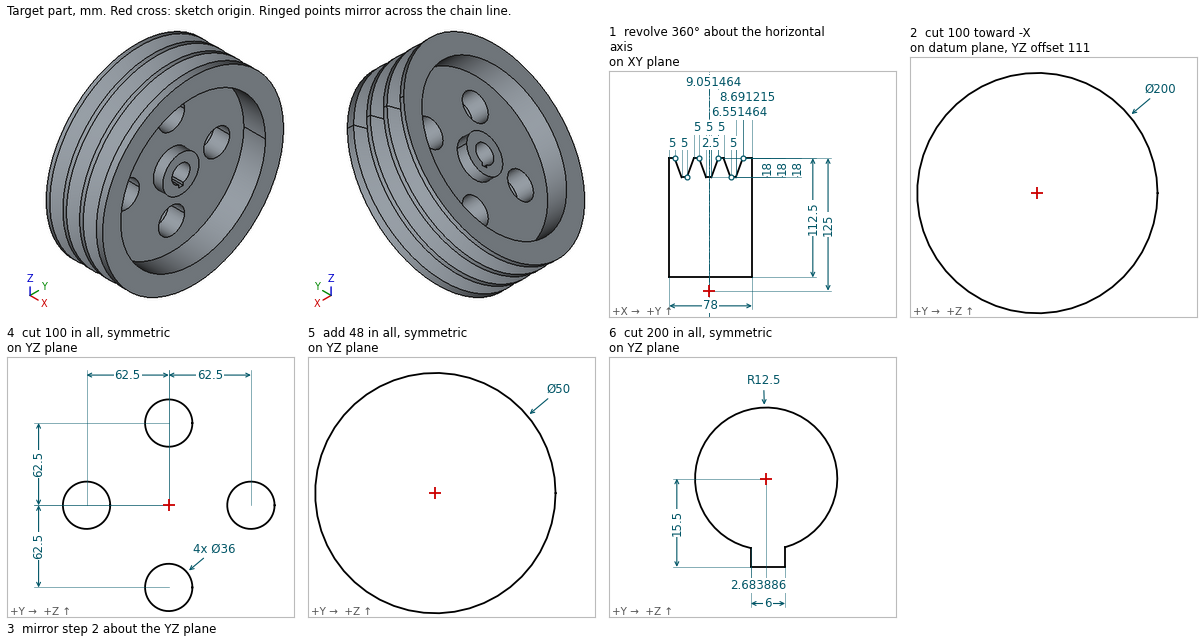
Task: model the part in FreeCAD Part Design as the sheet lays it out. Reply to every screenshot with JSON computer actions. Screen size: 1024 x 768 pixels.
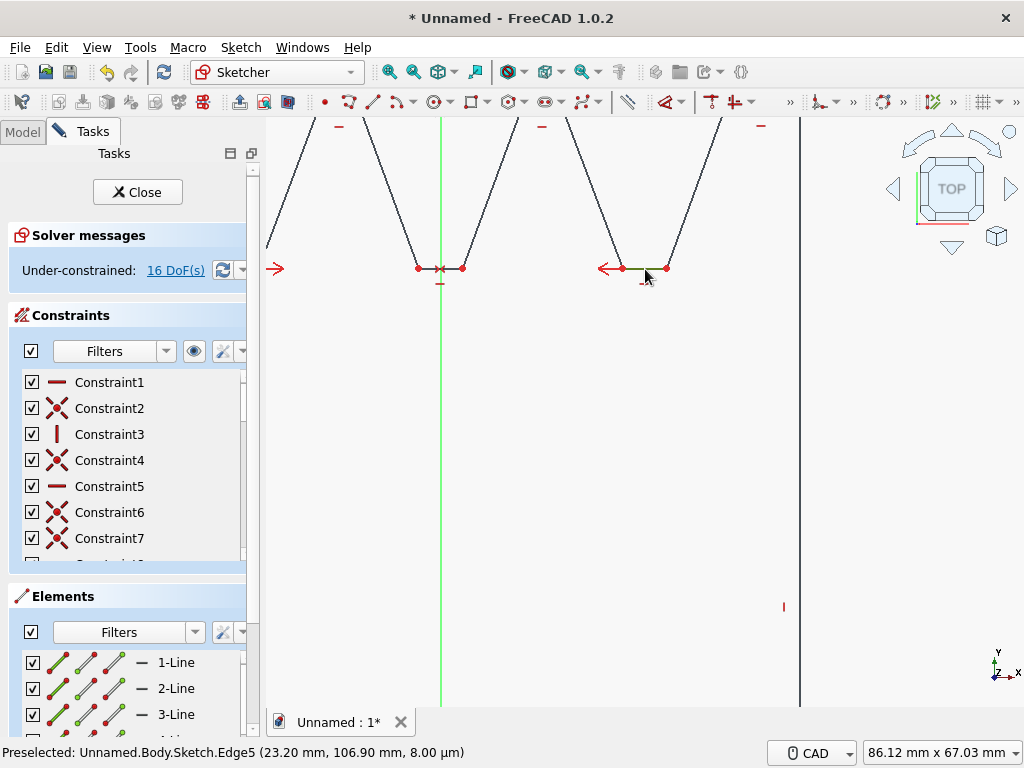
{"action": "left_click", "coordinate": [684, 102]}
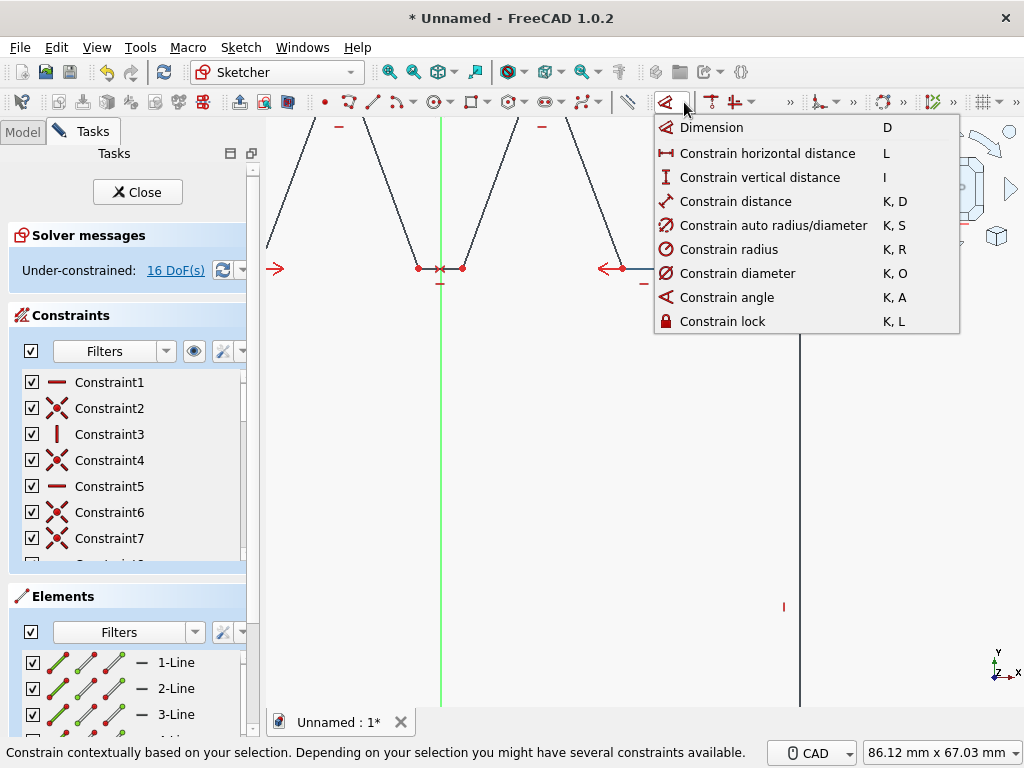
{"action": "left_click", "coordinate": [807, 153]}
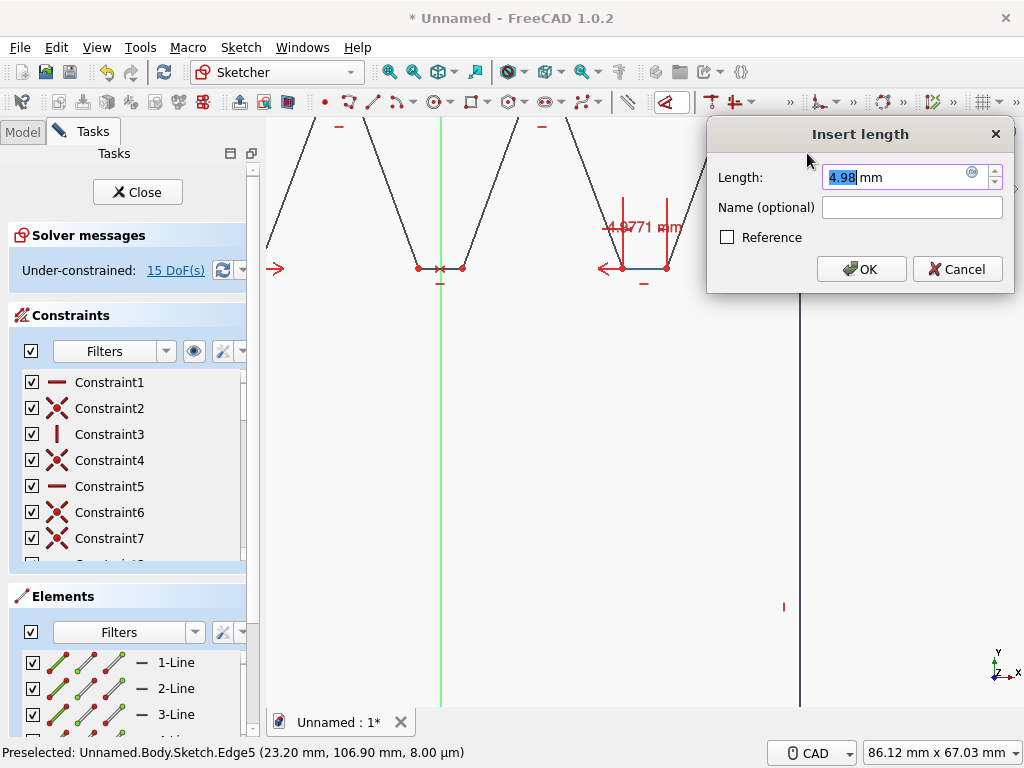
{"action": "type", "text": "5"}
{"action": "key", "text": "Return"}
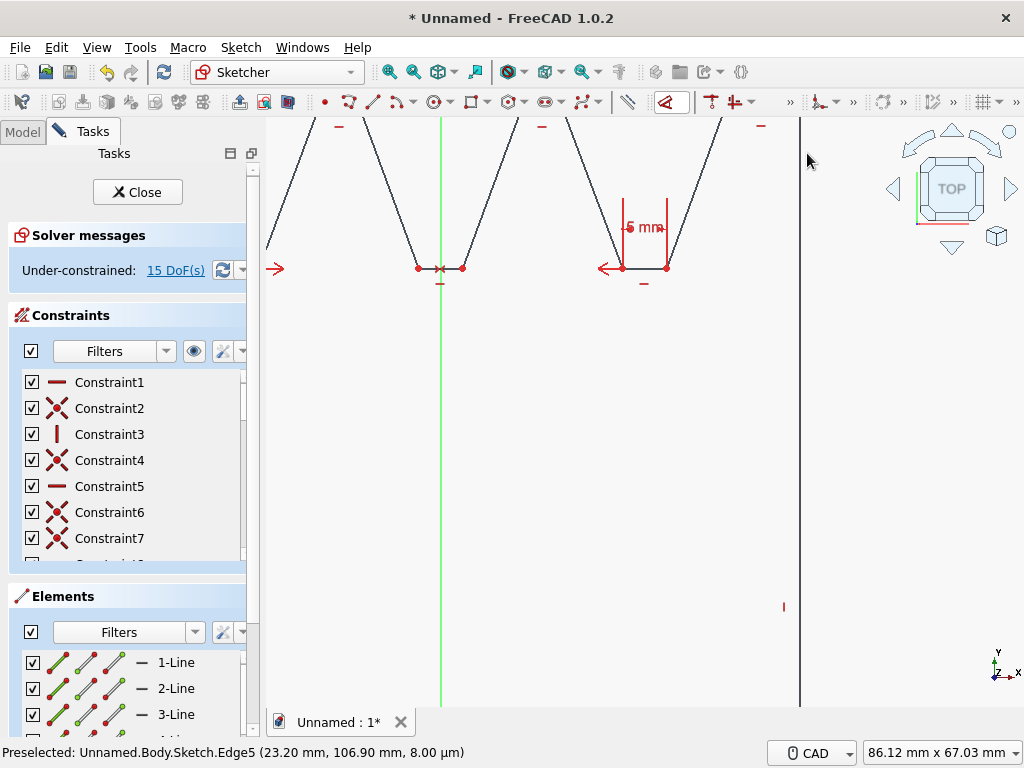
{"action": "scroll", "coordinate": [646, 268], "scroll_direction": "down", "scroll_amount": 5}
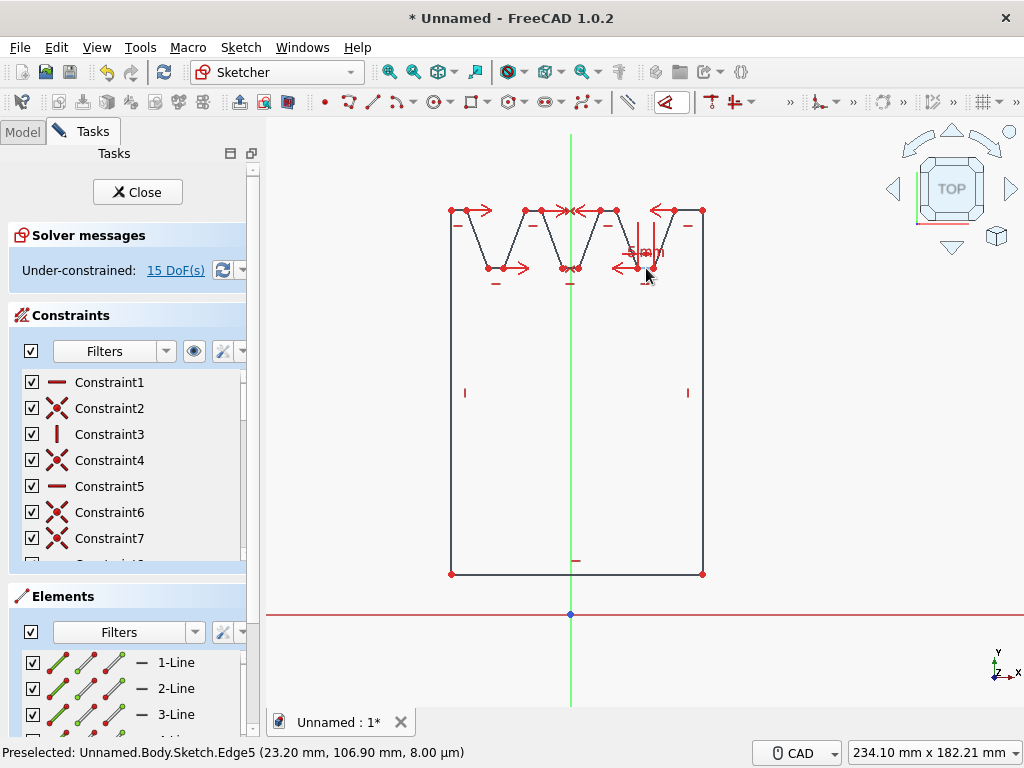
{"action": "scroll", "coordinate": [611, 211], "scroll_direction": "up", "scroll_amount": 6}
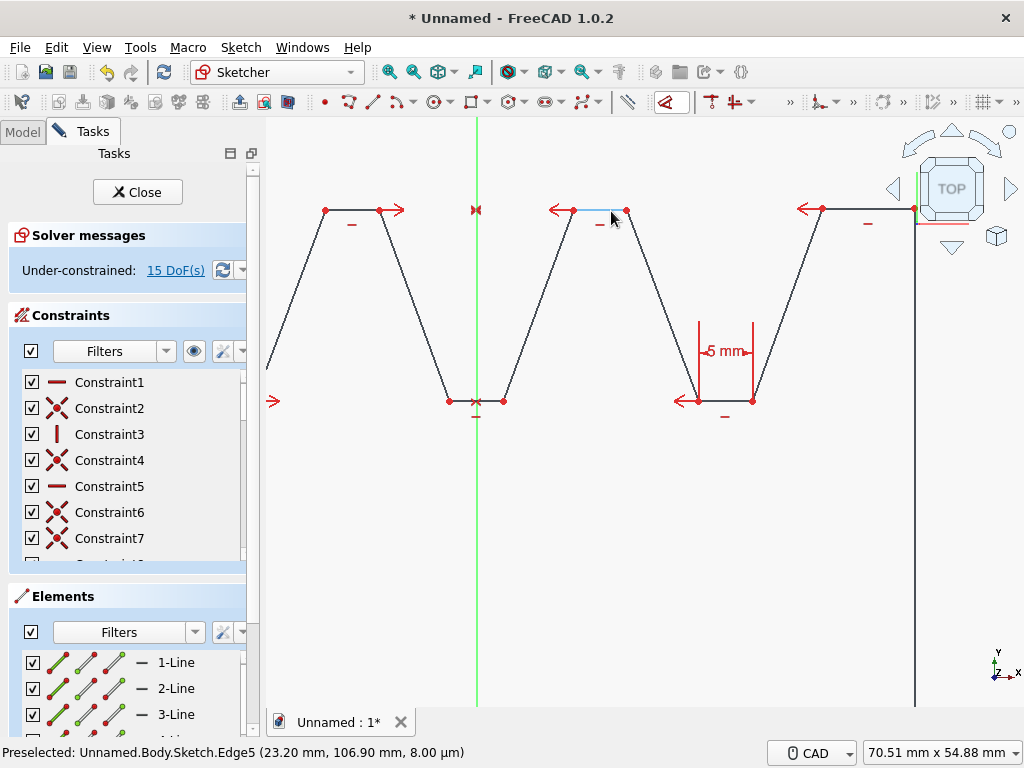
{"action": "left_click", "coordinate": [611, 210]}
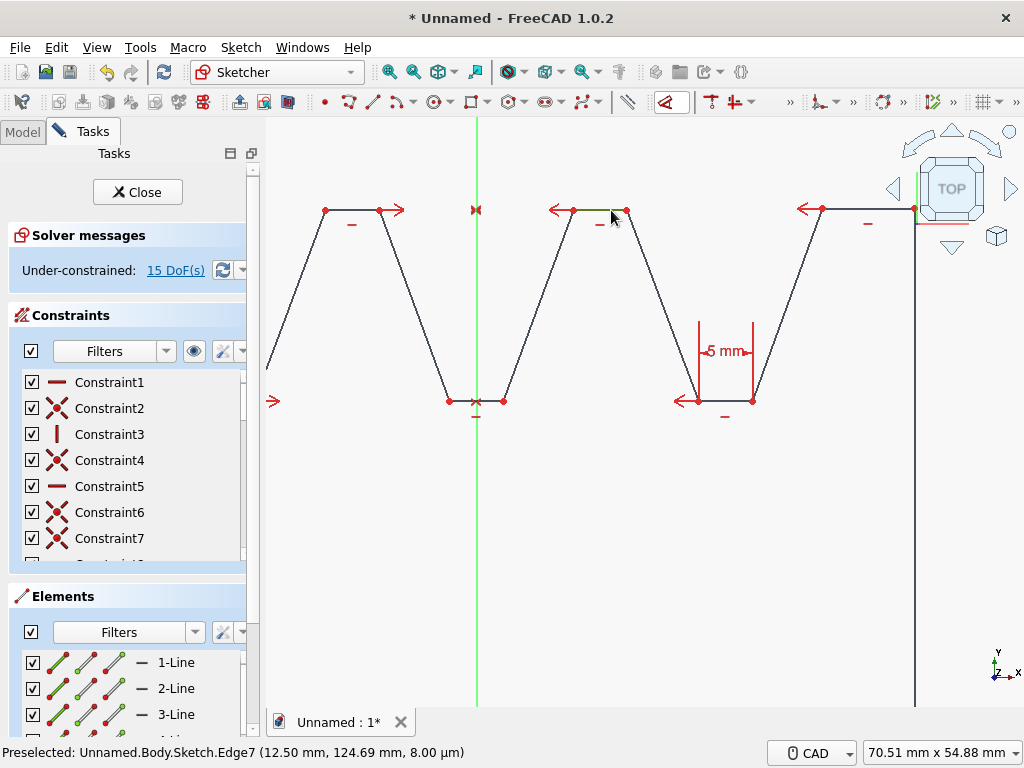
{"action": "left_click", "coordinate": [684, 102]}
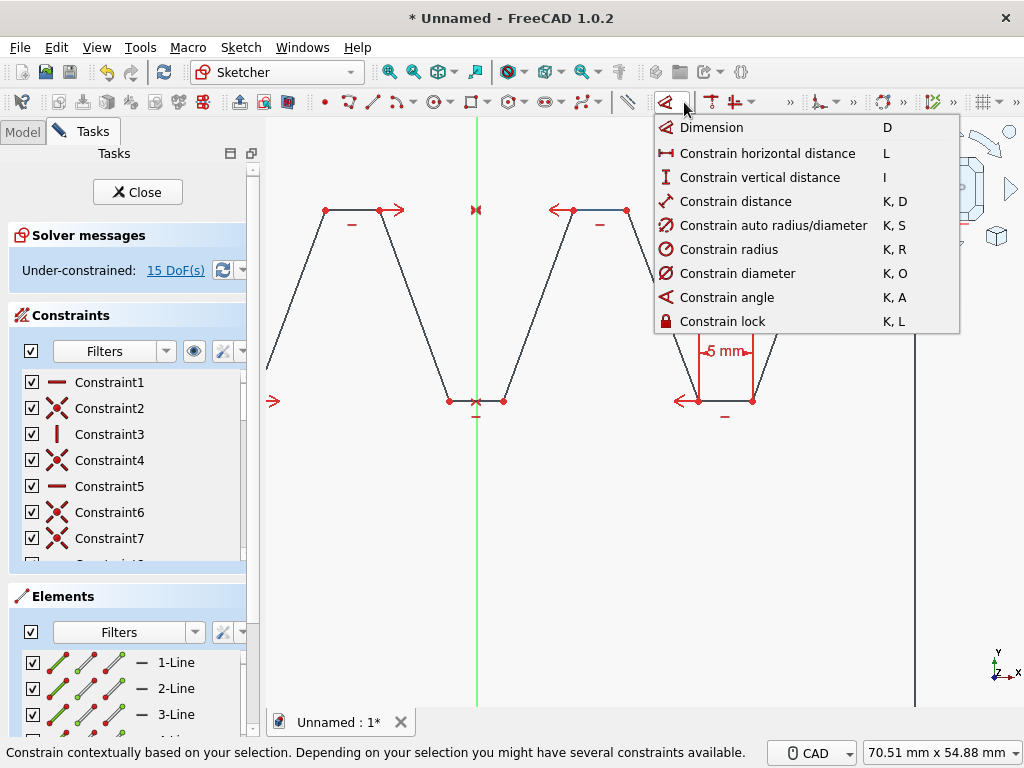
{"action": "left_click", "coordinate": [807, 153]}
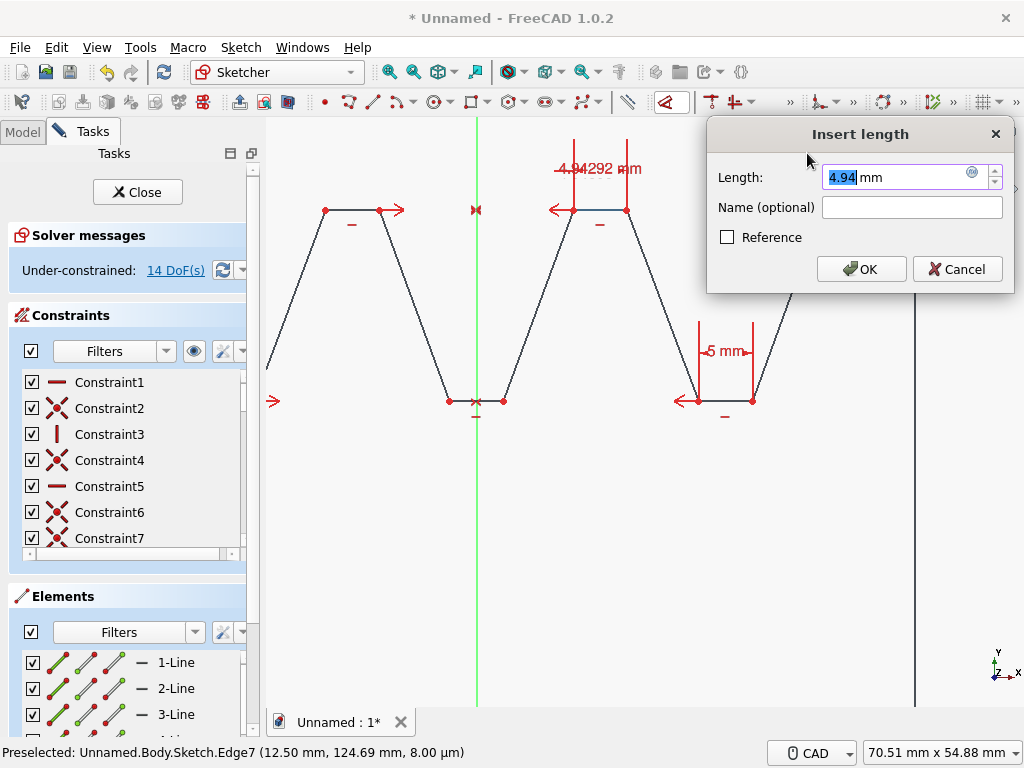
{"action": "type", "text": "5"}
{"action": "key", "text": "Return"}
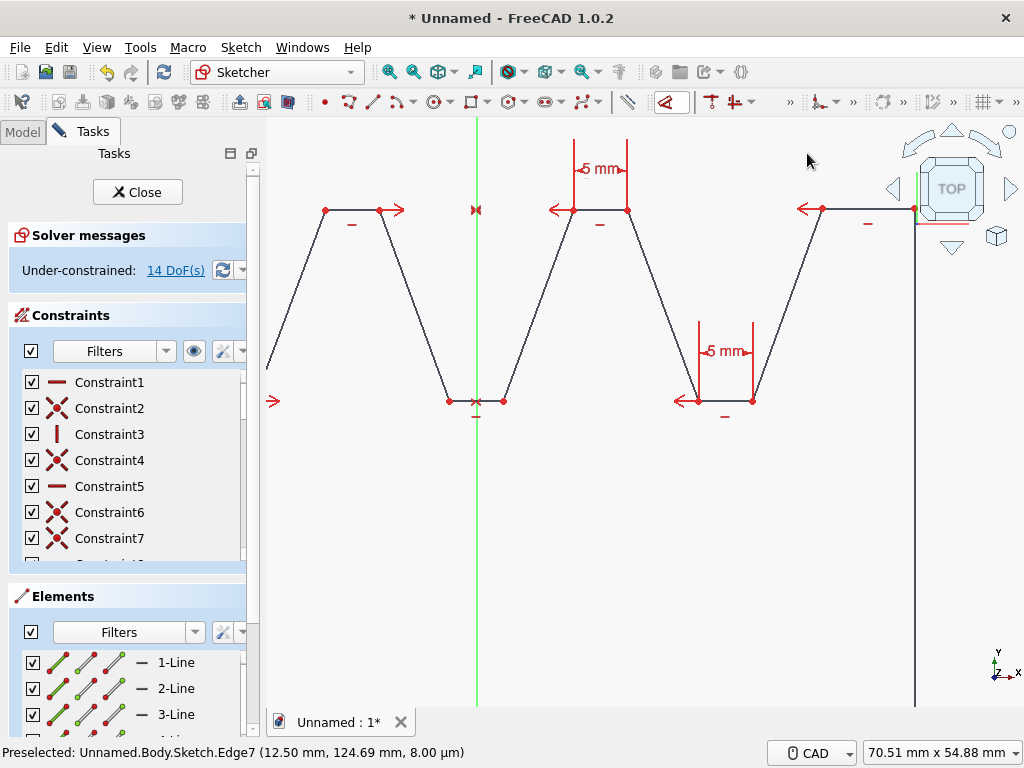
{"action": "scroll", "coordinate": [487, 401], "scroll_direction": "up", "scroll_amount": 2}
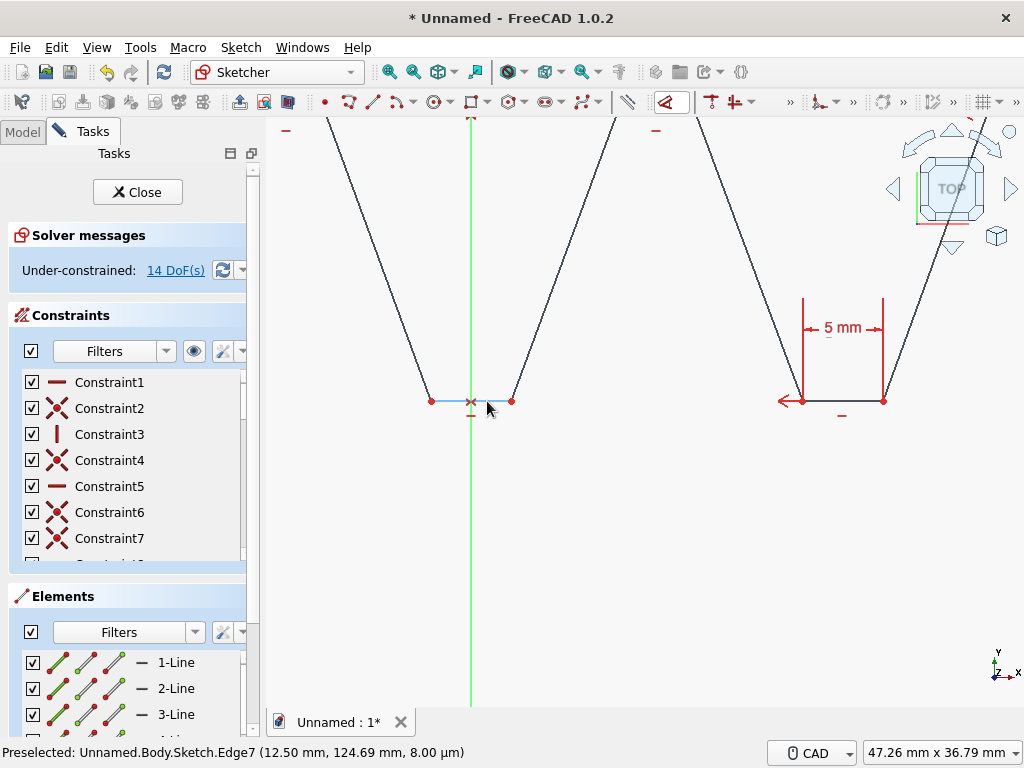
{"action": "left_click", "coordinate": [487, 401]}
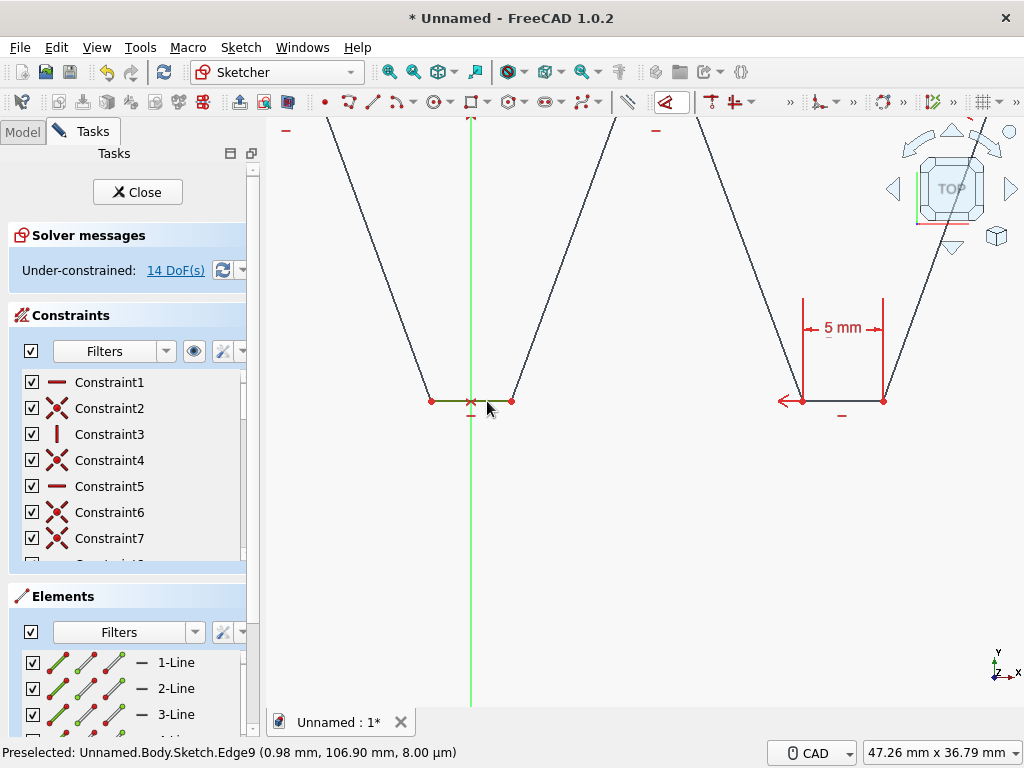
{"action": "left_click", "coordinate": [684, 102]}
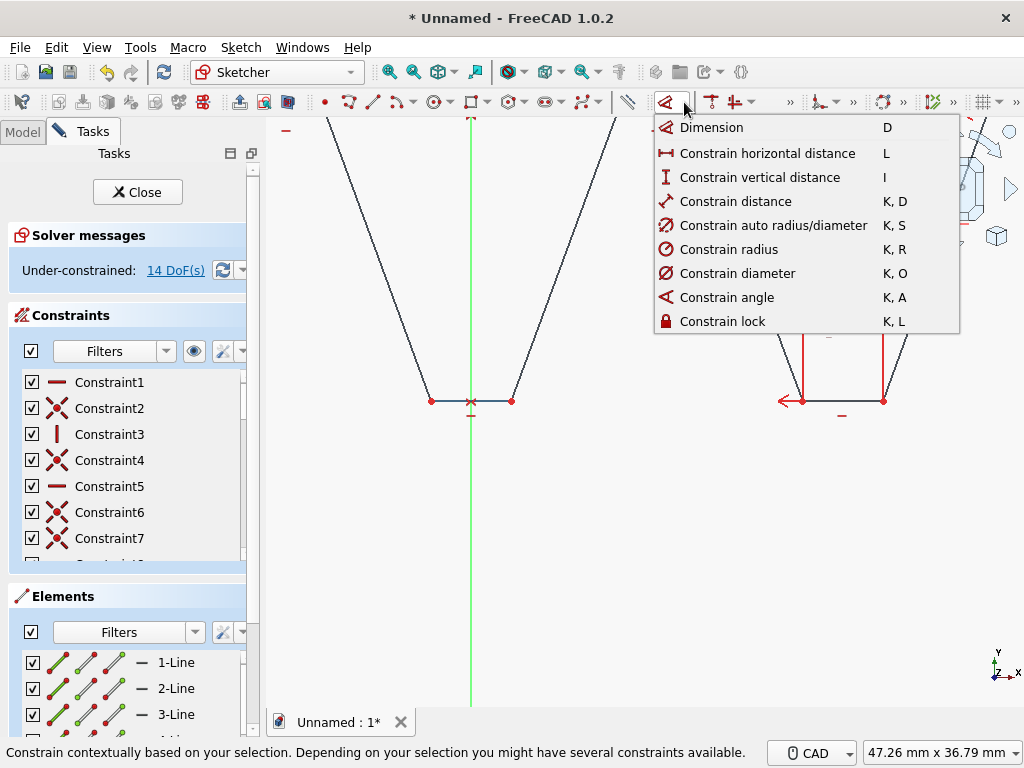
{"action": "left_click", "coordinate": [807, 153]}